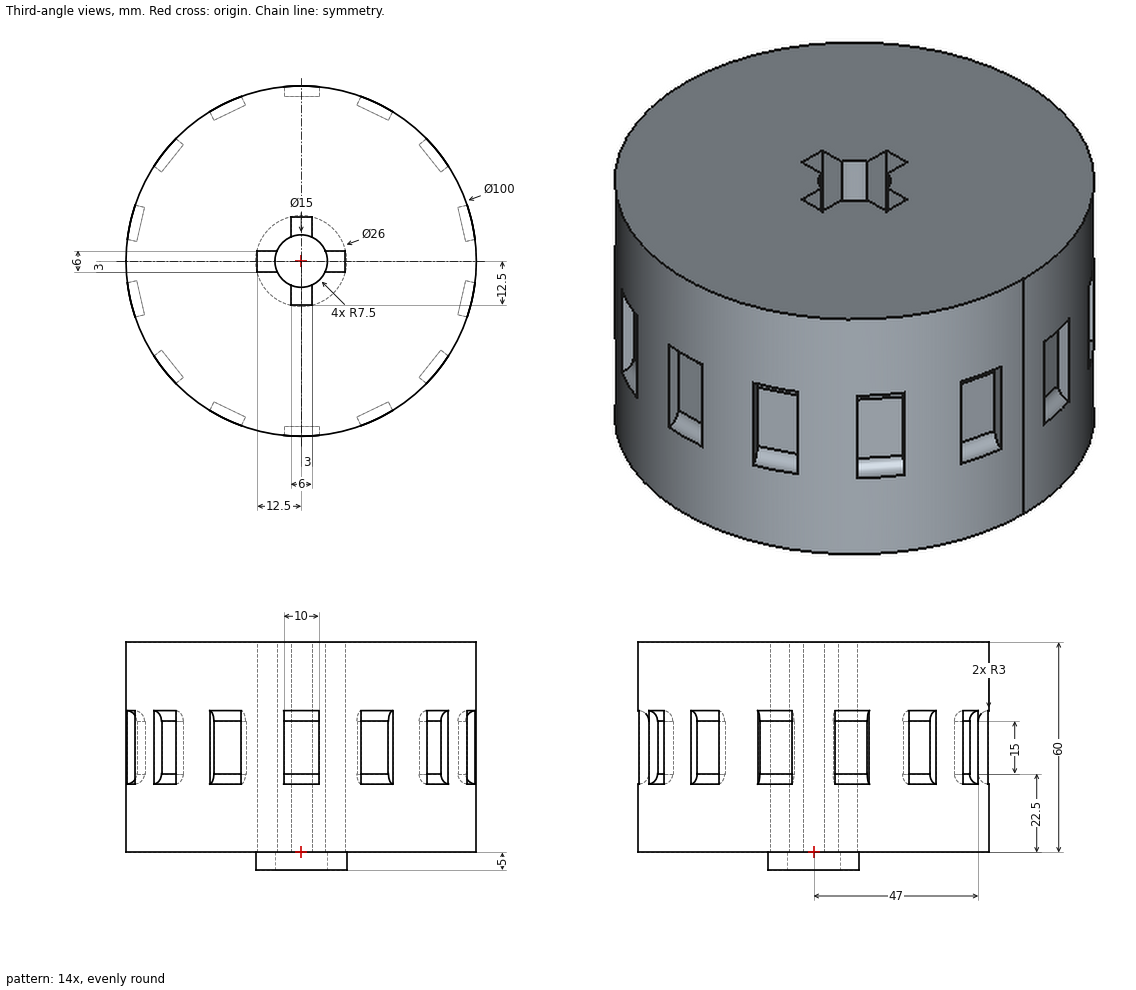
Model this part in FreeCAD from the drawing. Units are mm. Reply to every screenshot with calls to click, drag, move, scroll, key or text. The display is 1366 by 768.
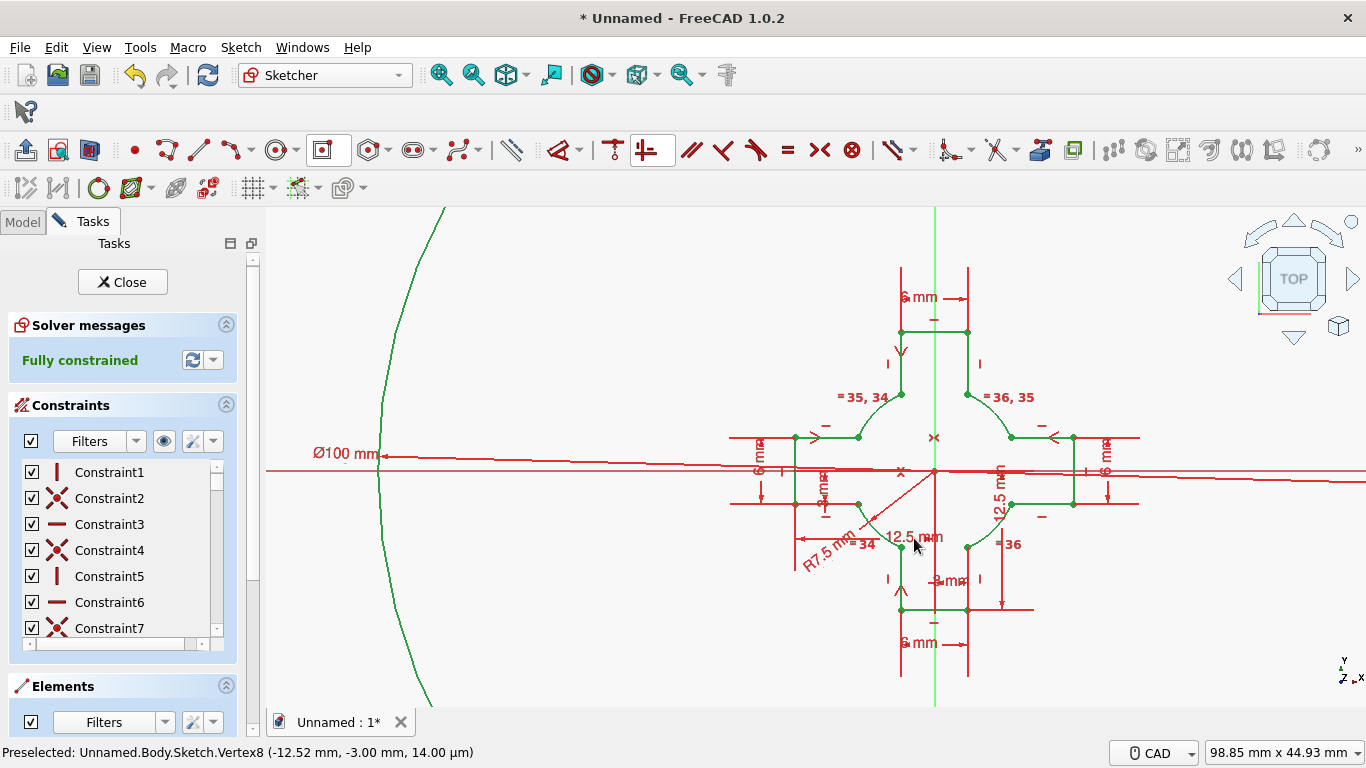
click(123, 282)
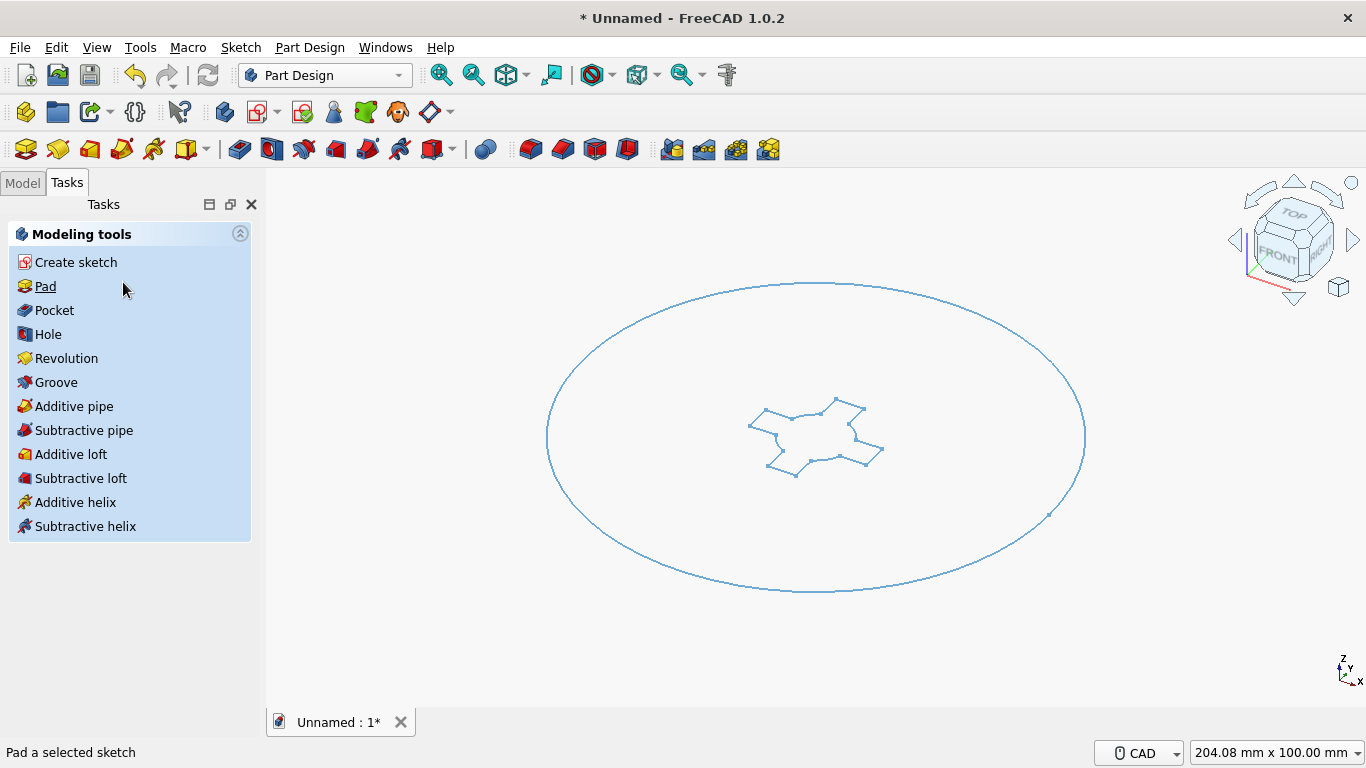
click(26, 150)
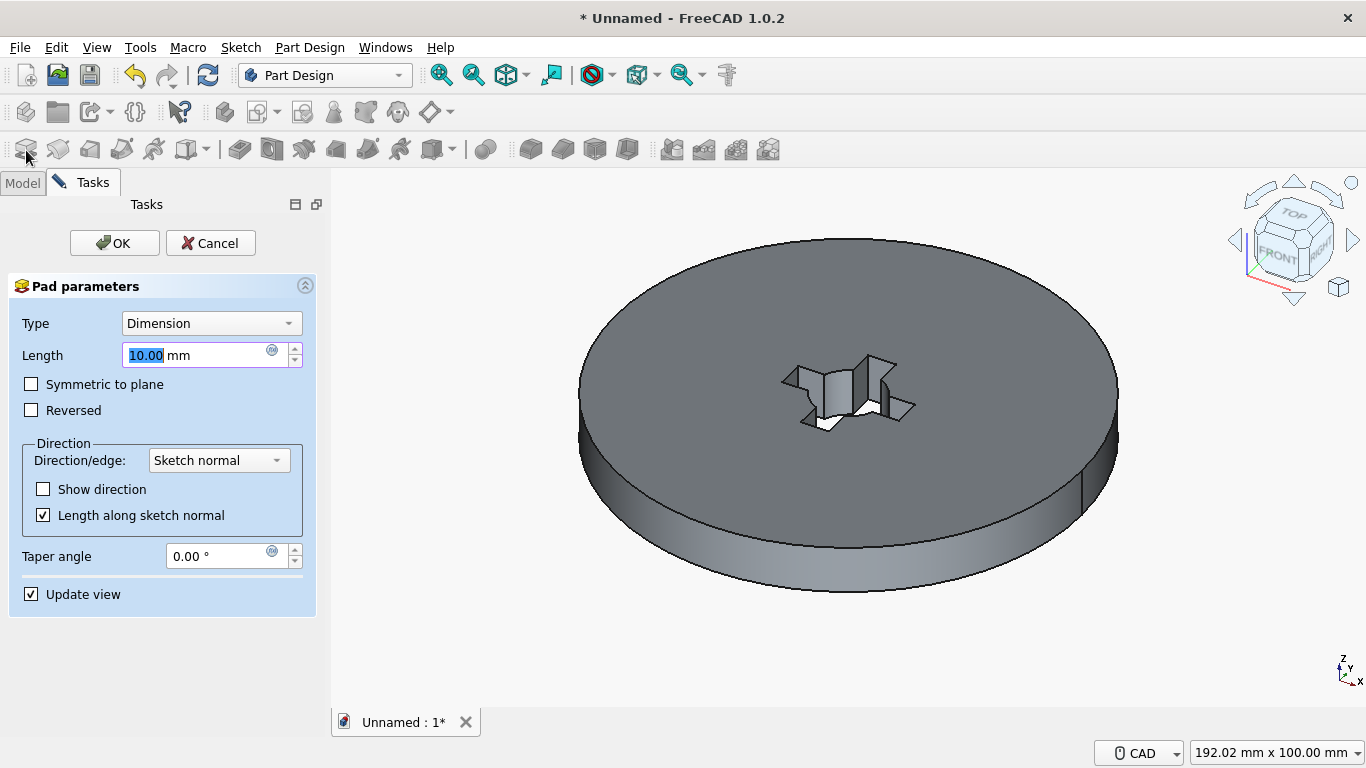
text(60)
key(Tab)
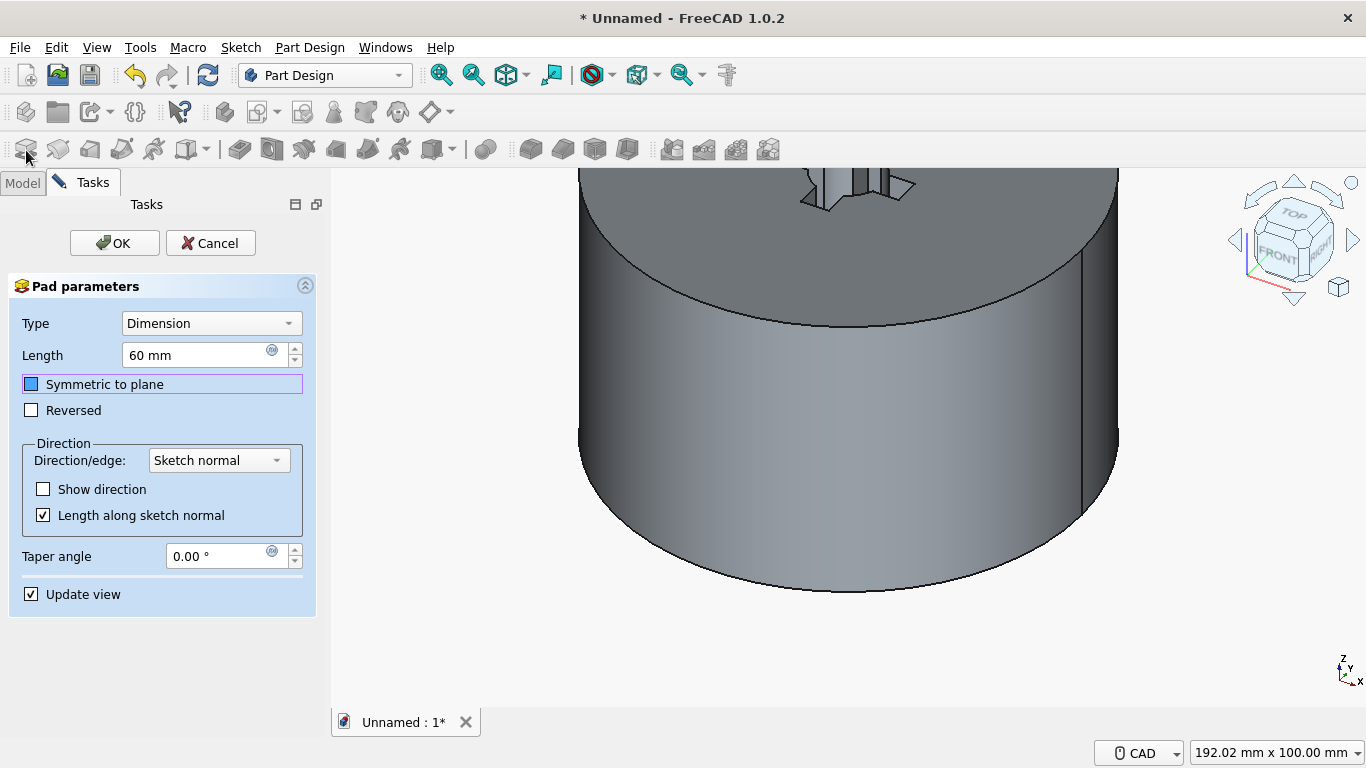
click(115, 243)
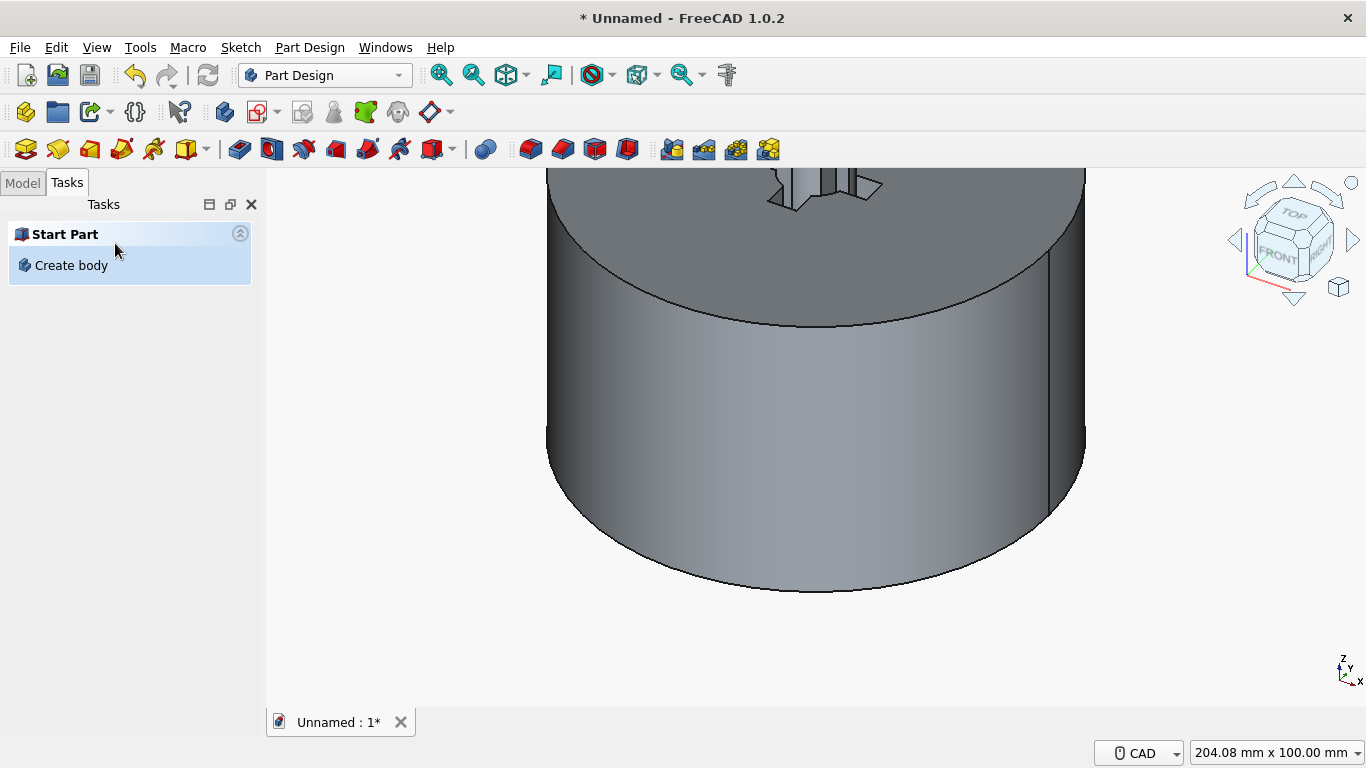
key(v)
key(f)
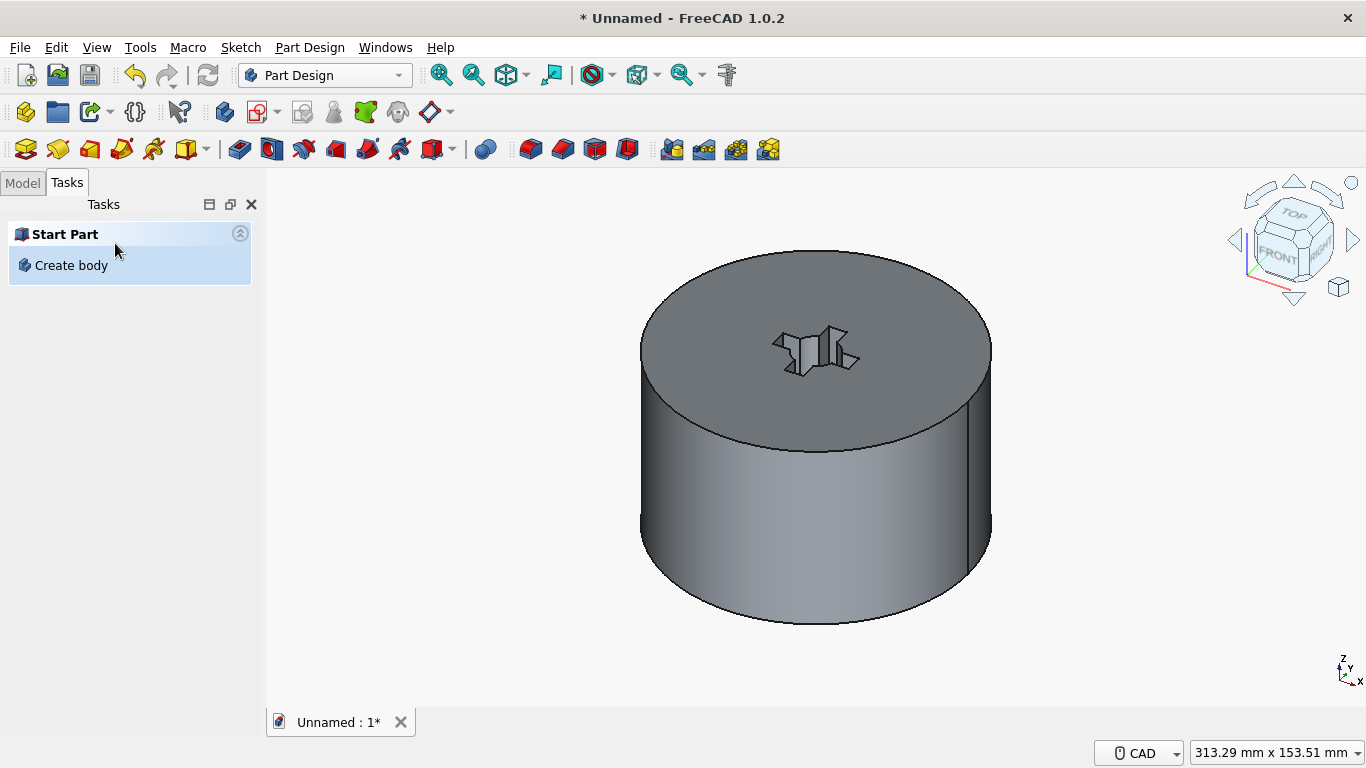
click(23, 182)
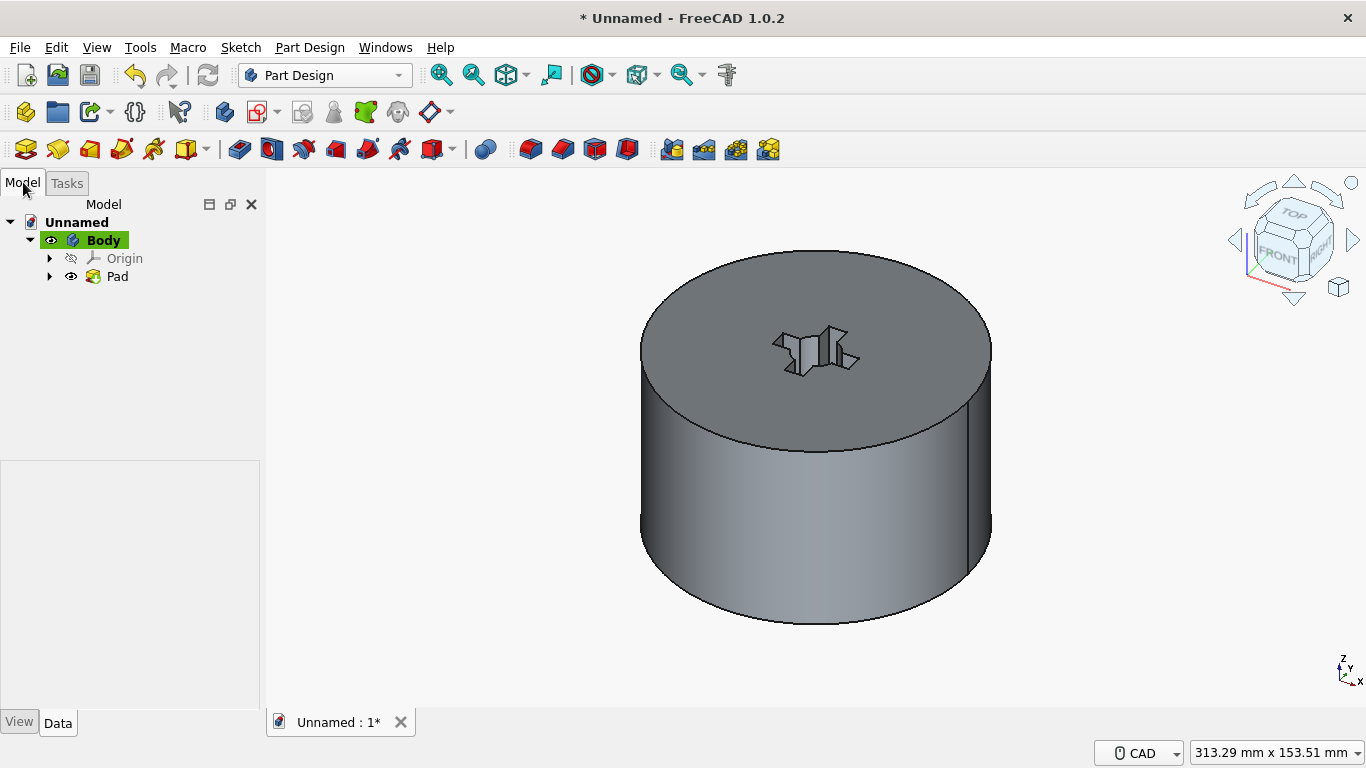
click(50, 258)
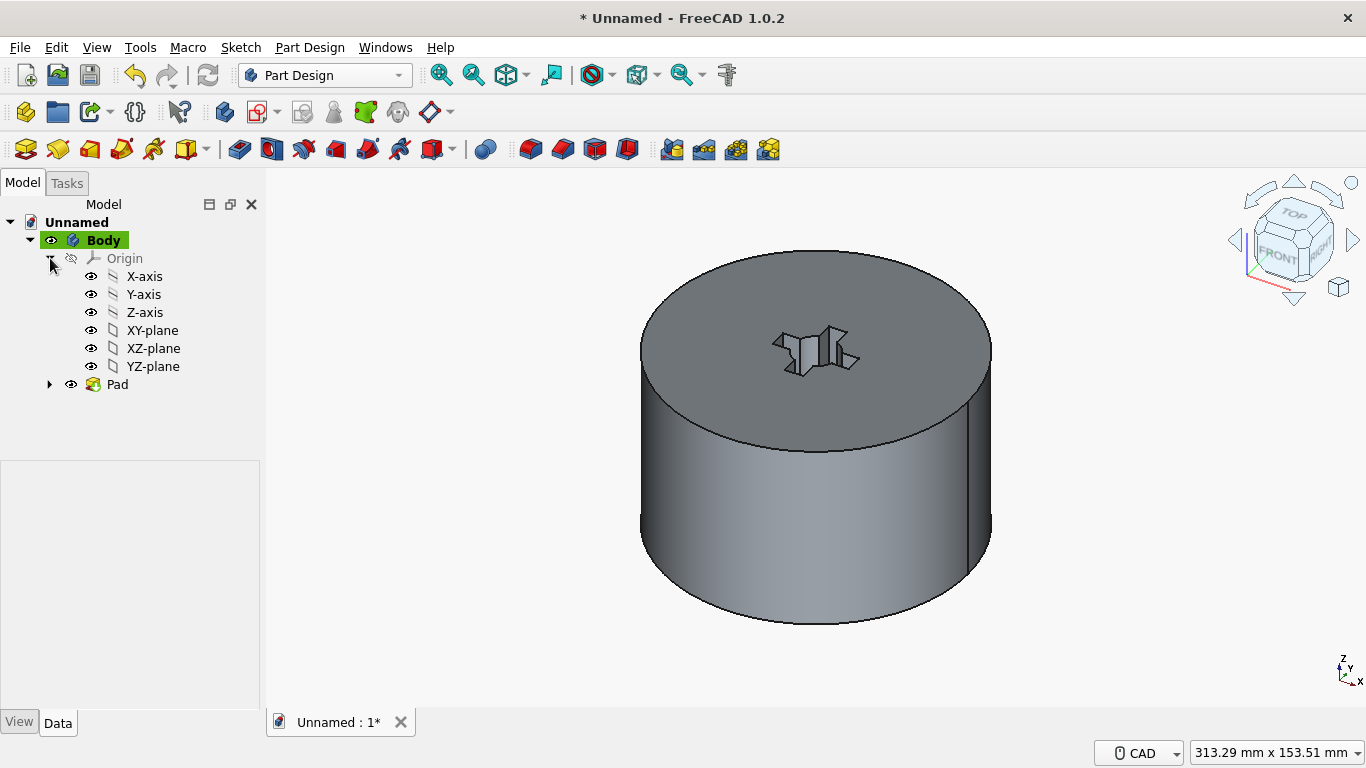
click(136, 330)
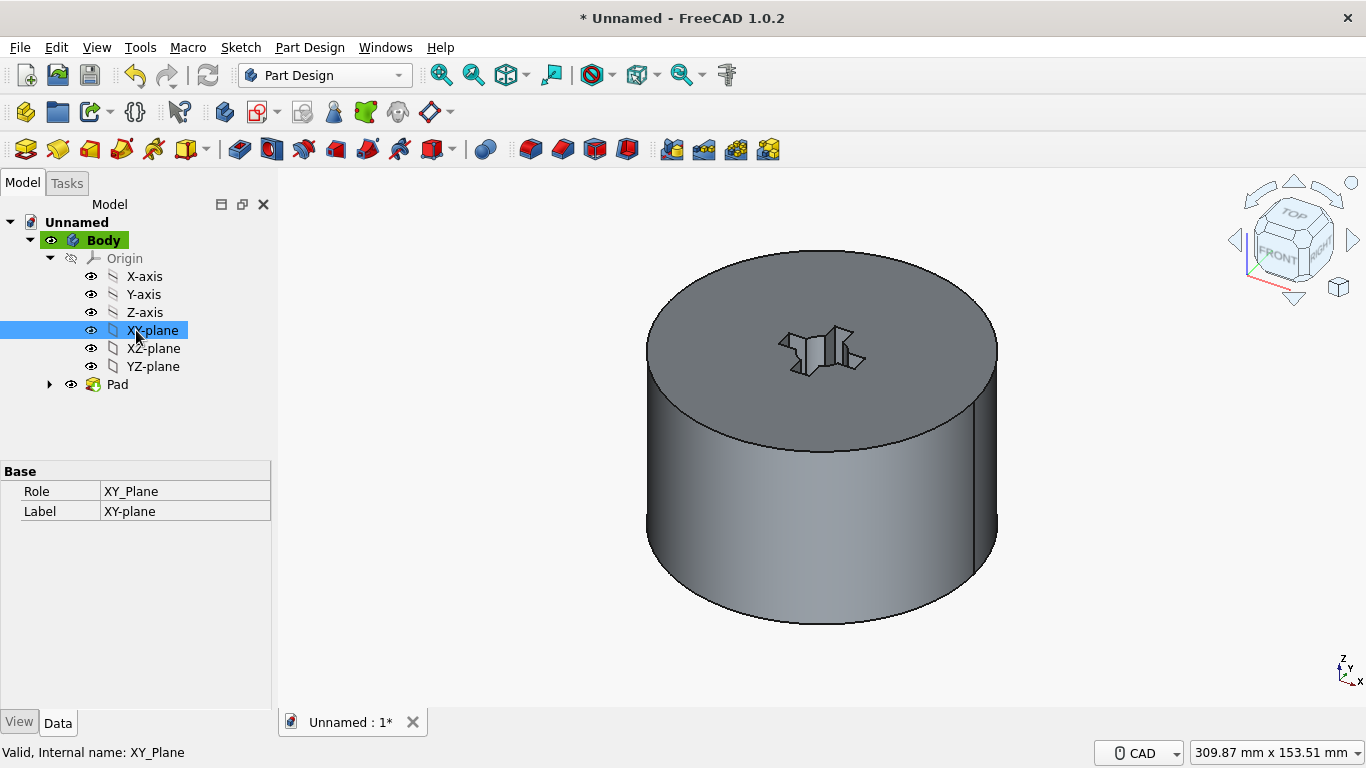
click(430, 112)